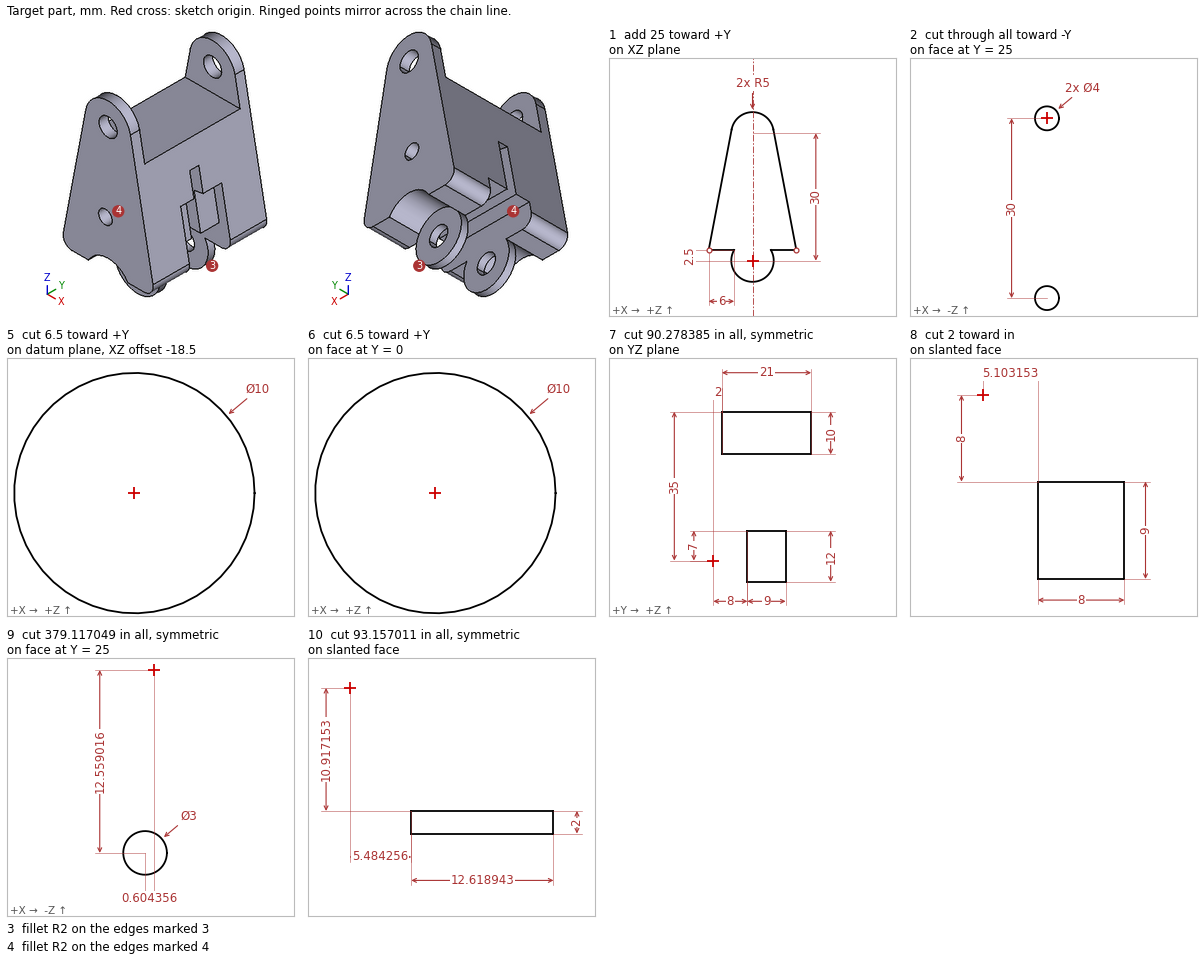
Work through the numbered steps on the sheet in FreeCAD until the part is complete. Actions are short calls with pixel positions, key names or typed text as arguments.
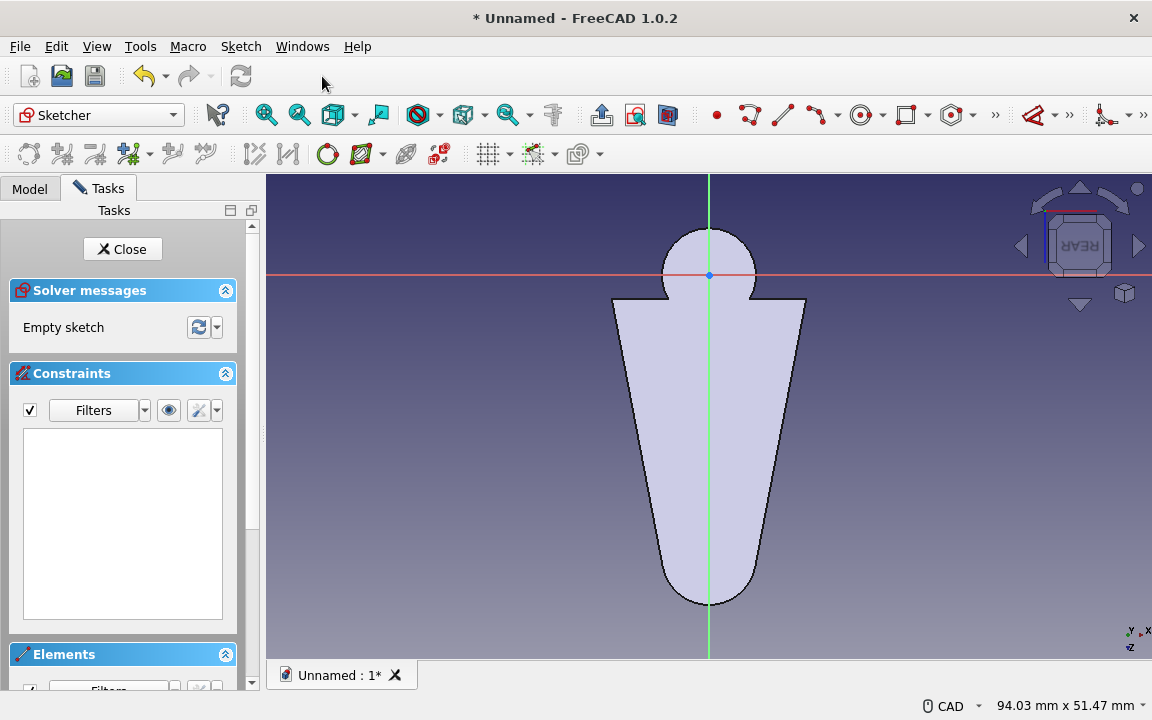
key(g)
key(c)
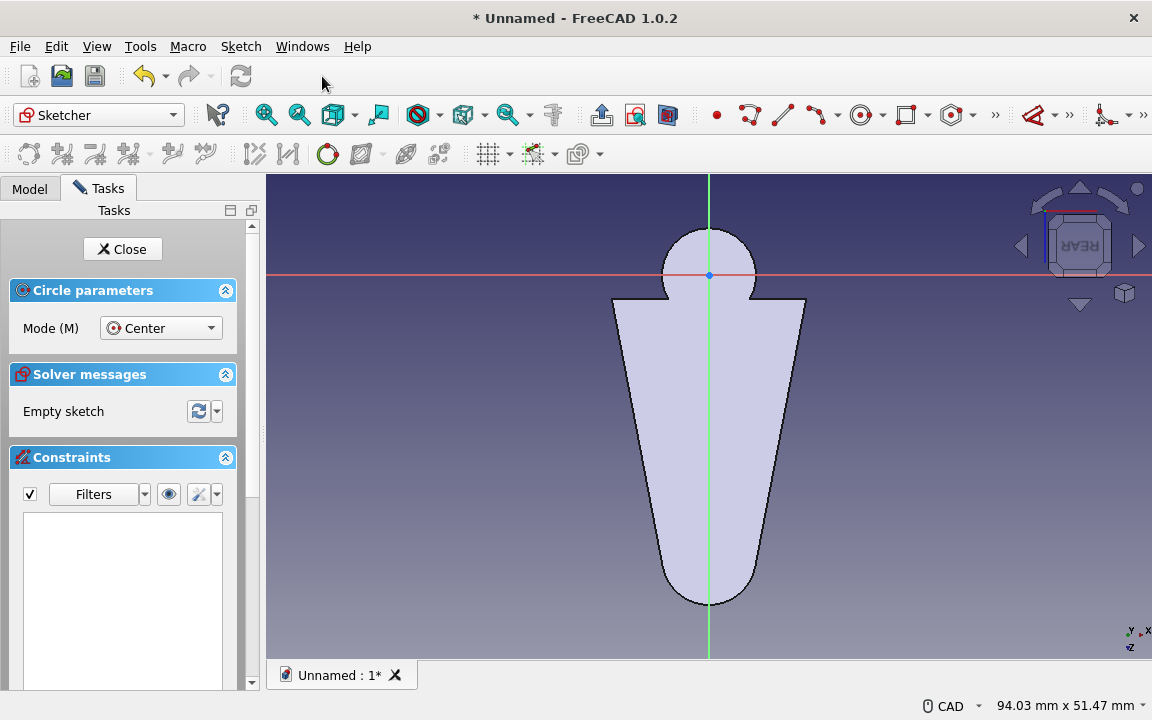
click(709, 275)
move(722, 262)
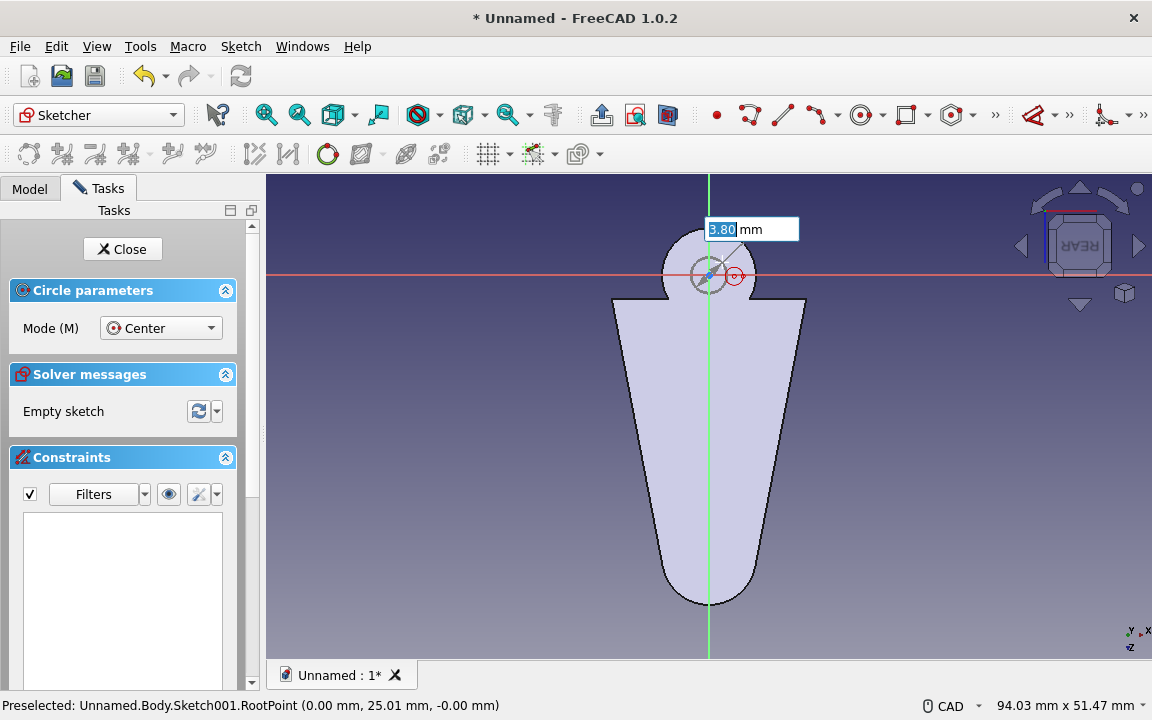
text(4)
key(Return)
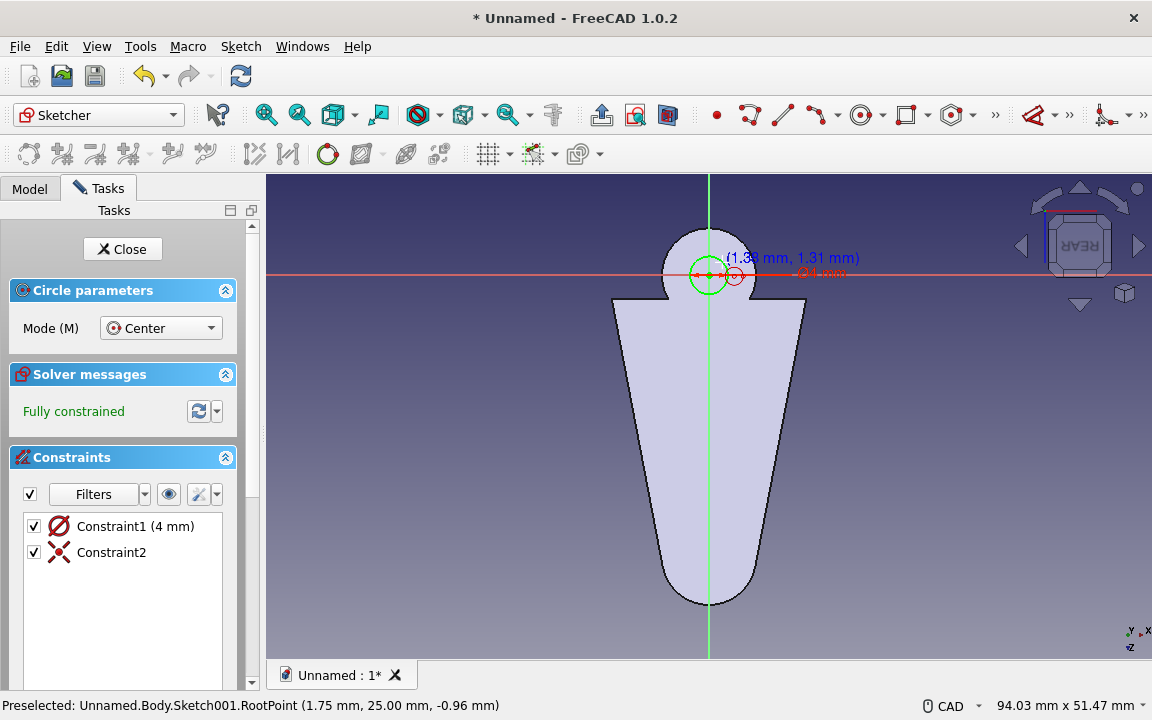
click(709, 558)
move(727, 552)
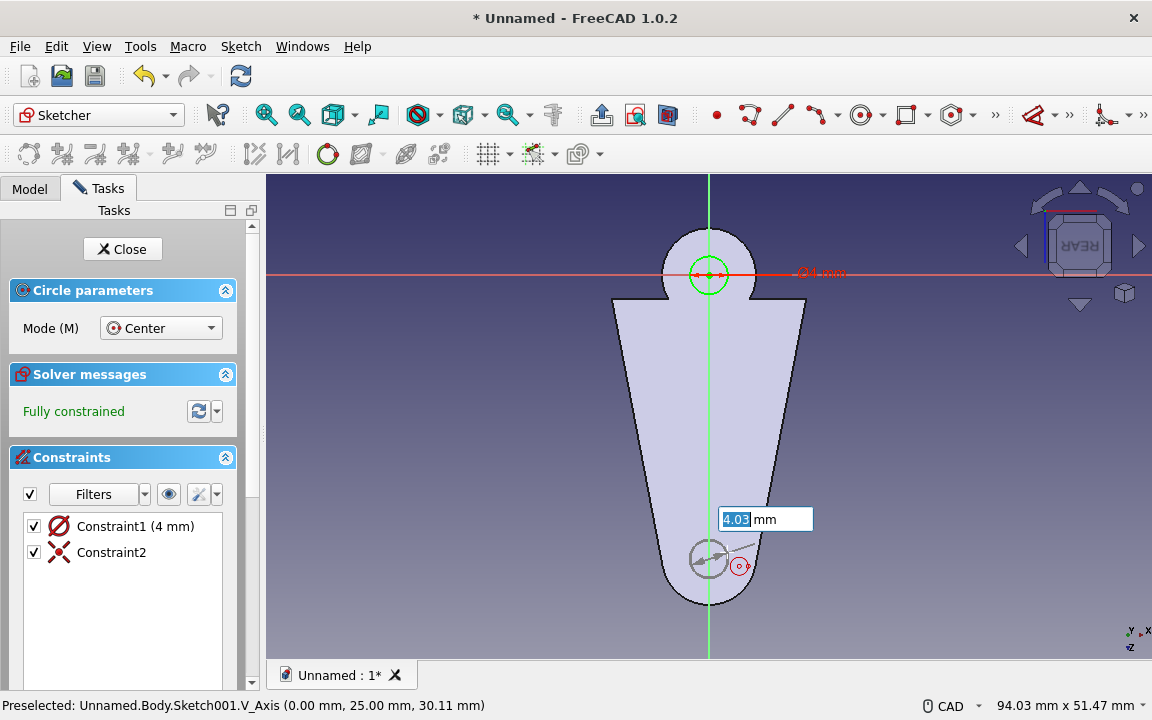
text(4)
key(Return)
key(Escape)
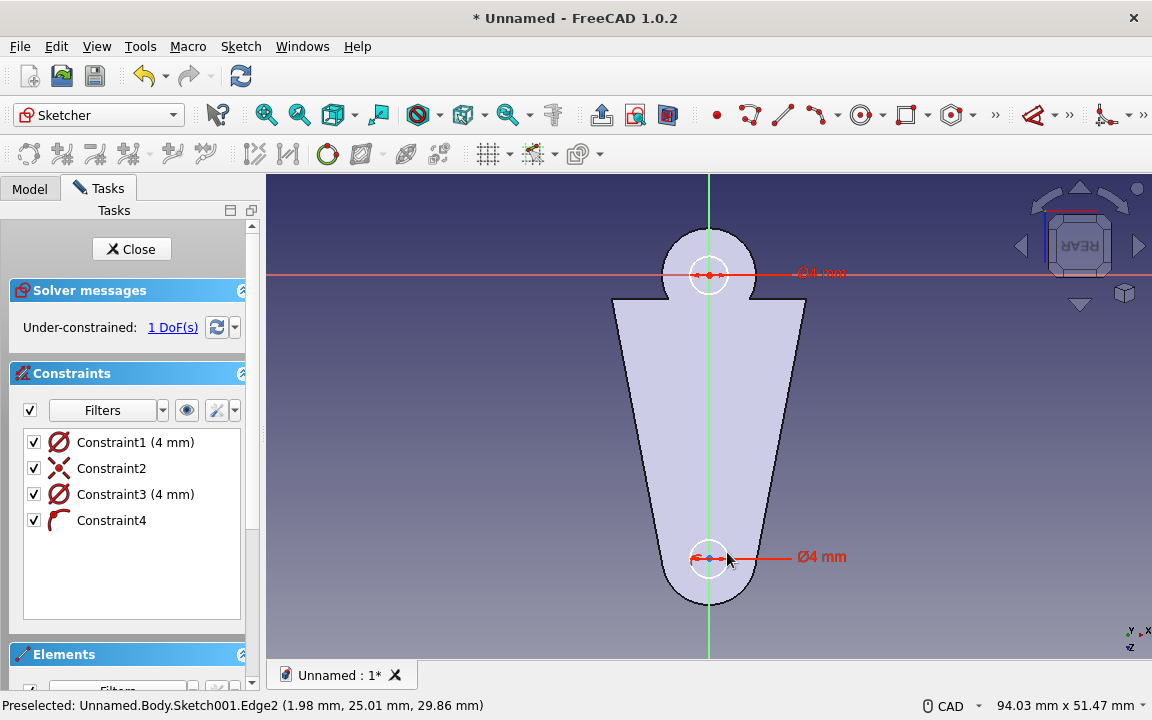
click(1032, 116)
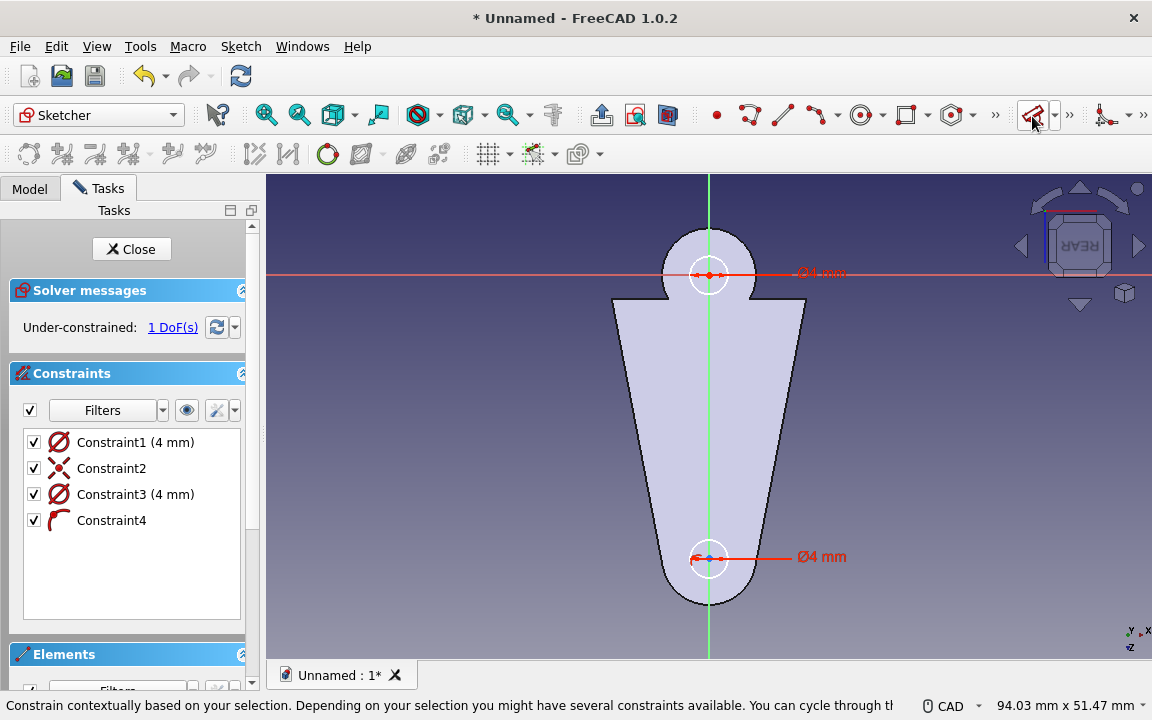
click(709, 559)
click(743, 417)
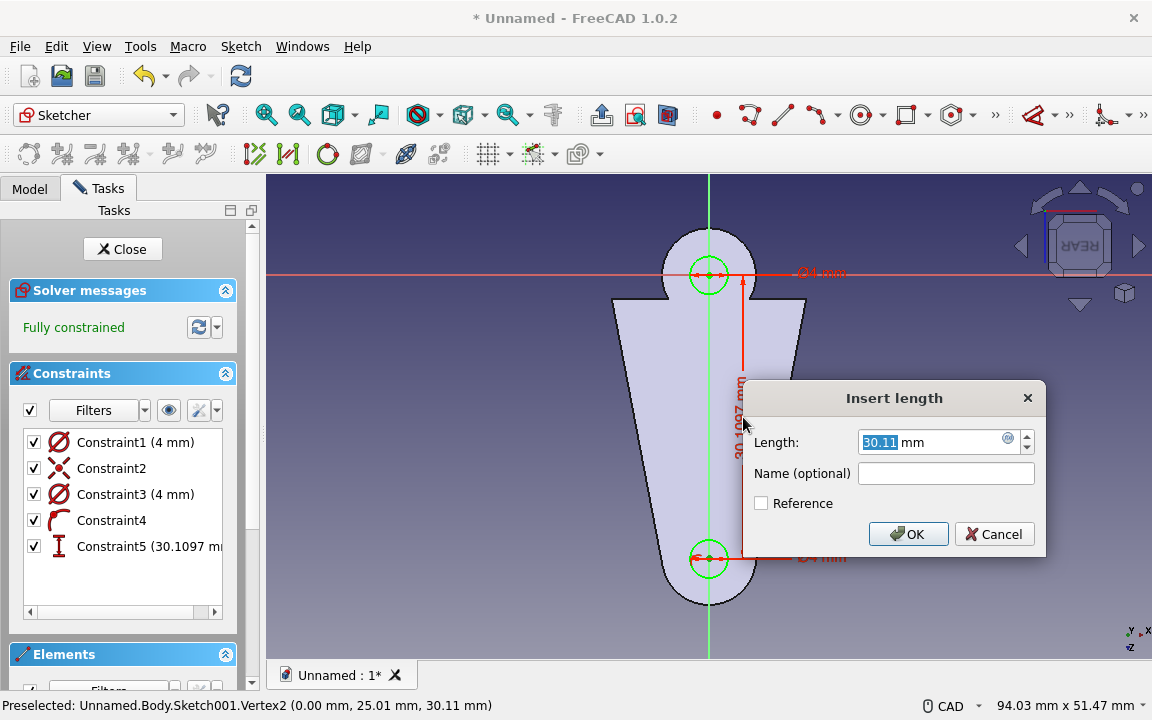
text(30)
key(Return)
key(Escape)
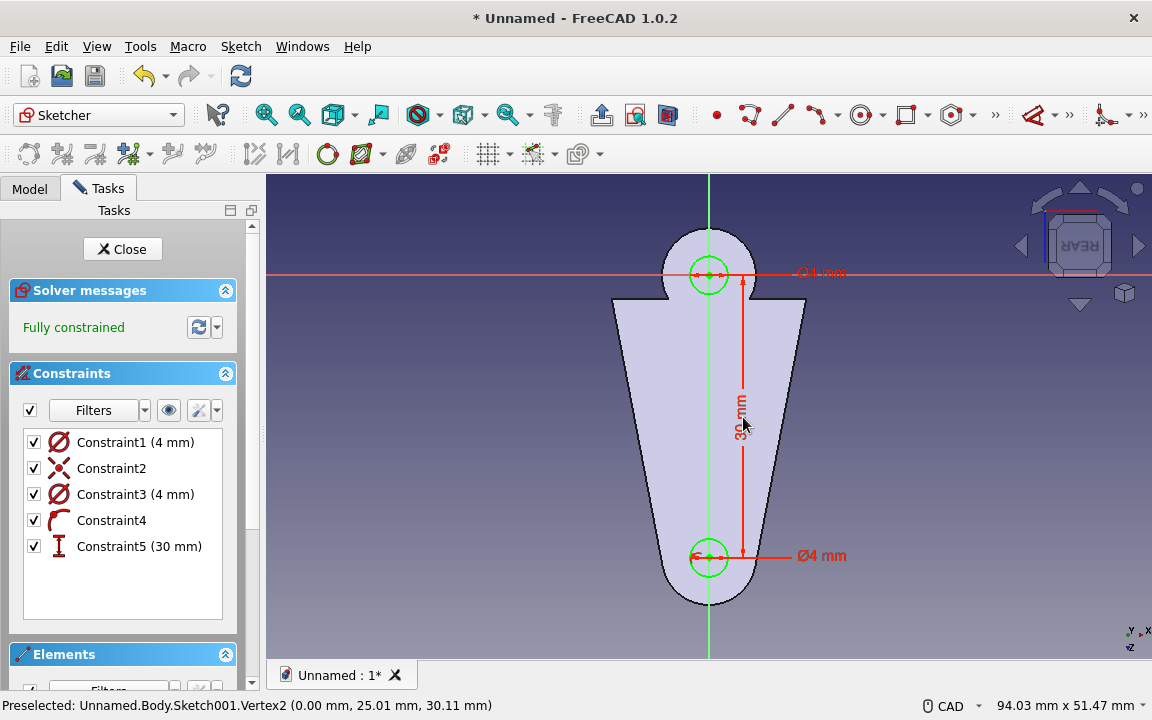
click(123, 249)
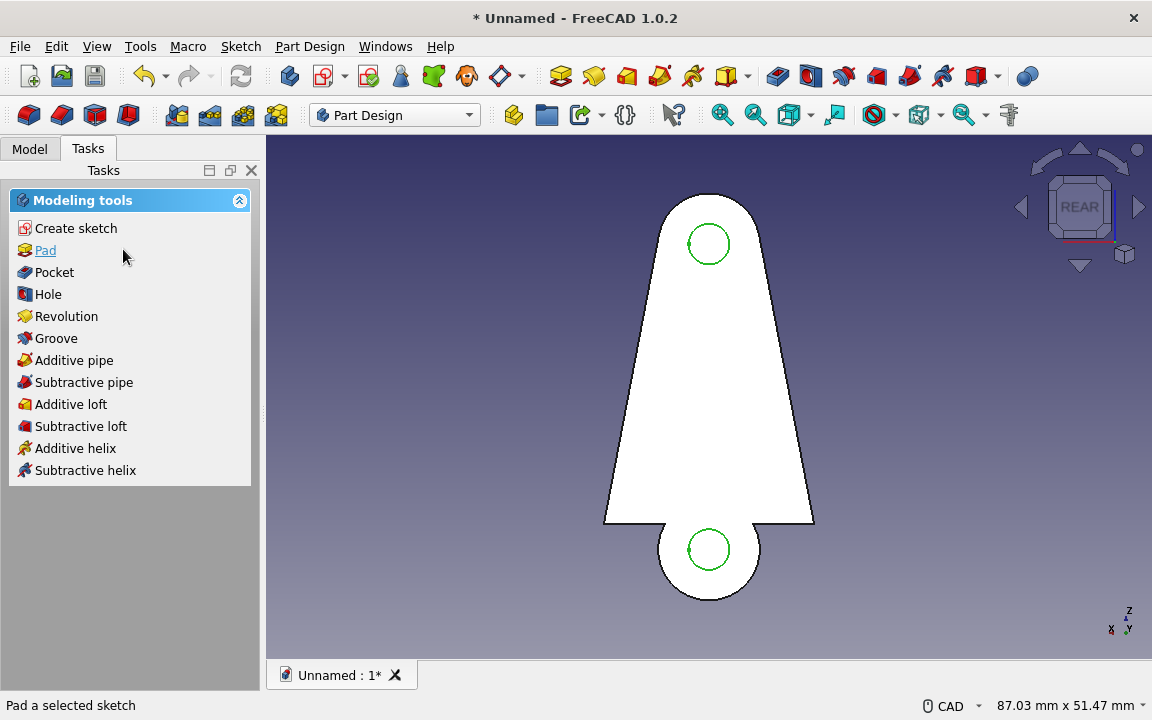
click(778, 76)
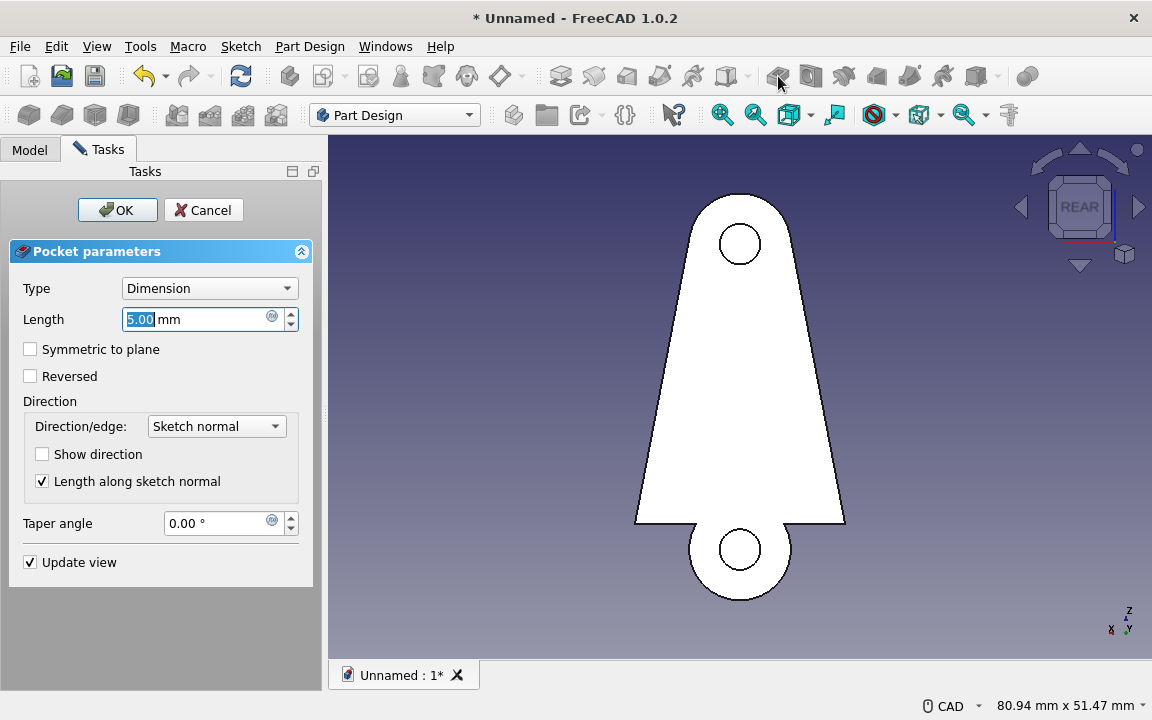
click(210, 288)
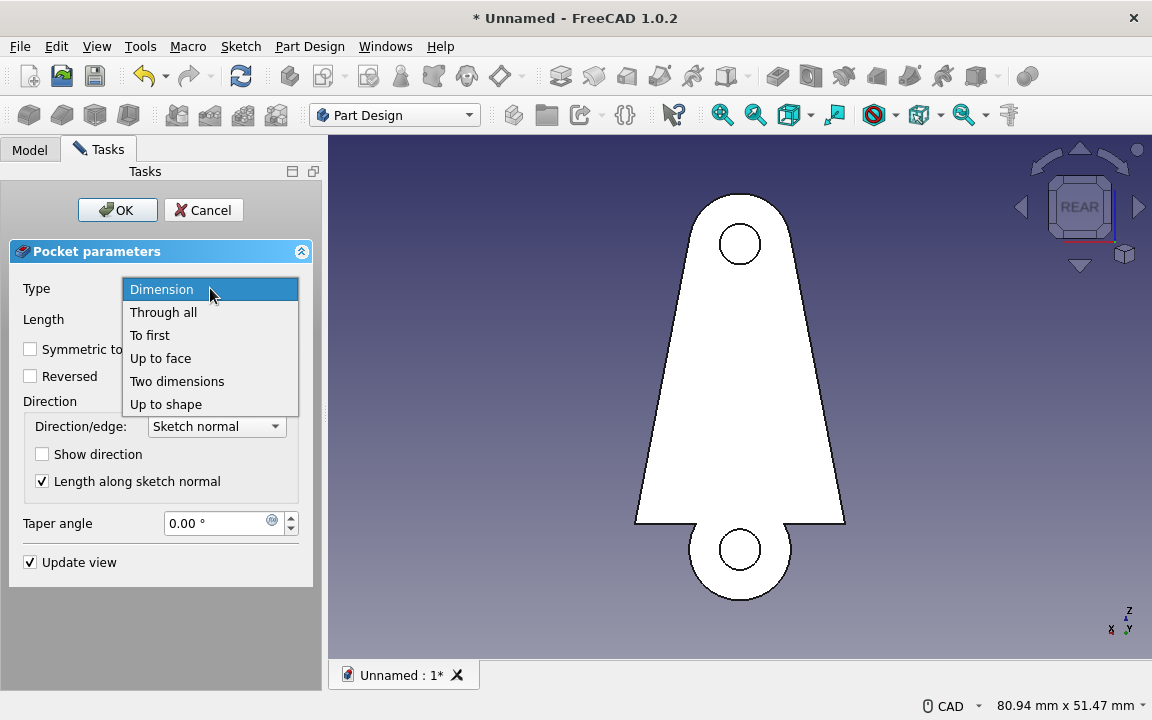
click(208, 312)